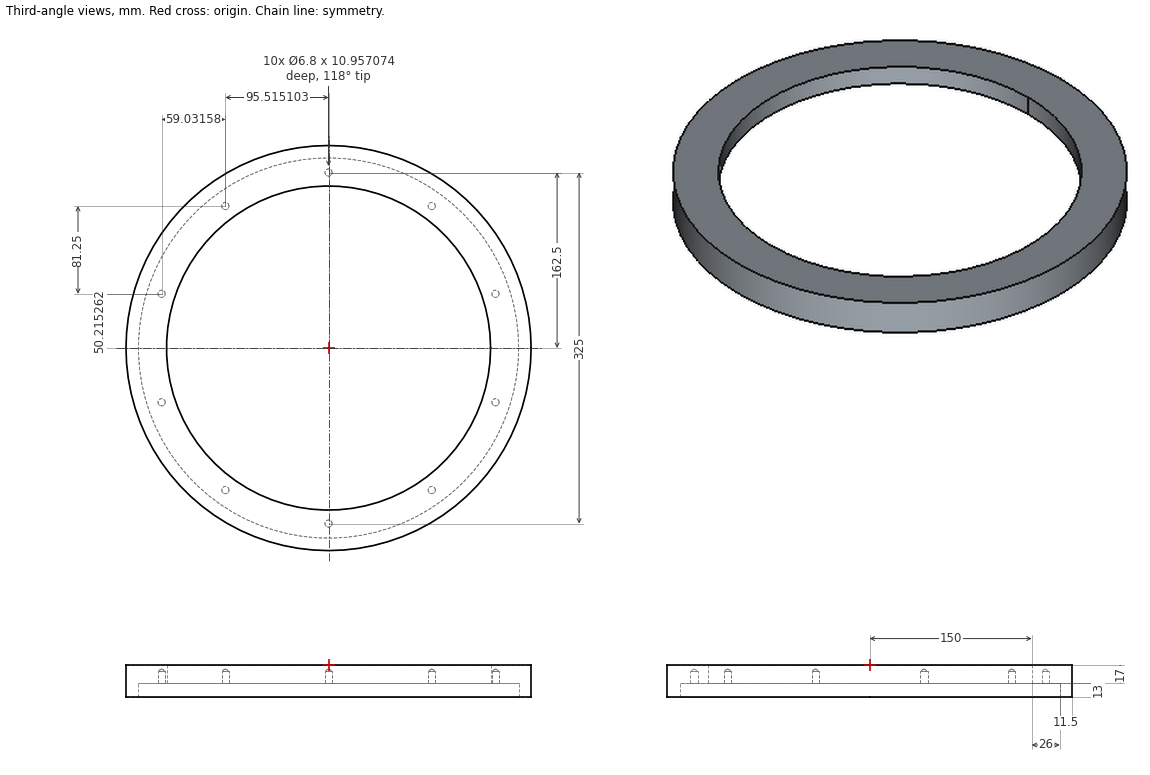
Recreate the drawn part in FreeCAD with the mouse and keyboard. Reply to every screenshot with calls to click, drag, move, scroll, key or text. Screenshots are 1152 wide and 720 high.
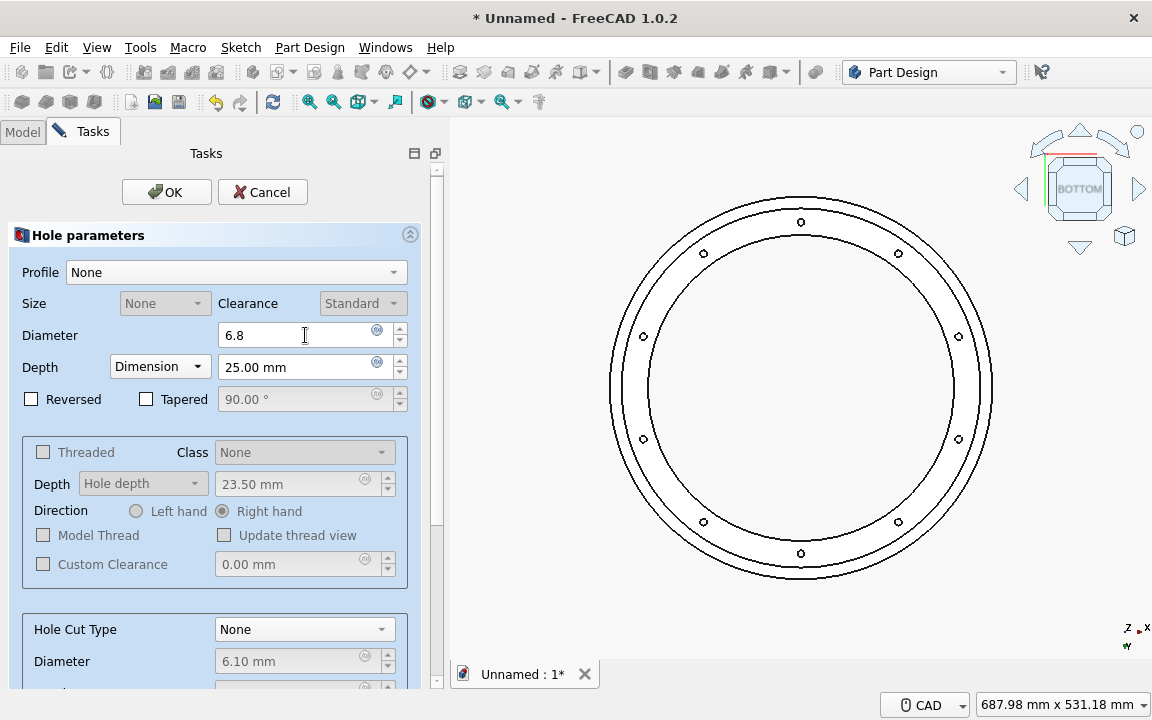
triple_click(305, 367)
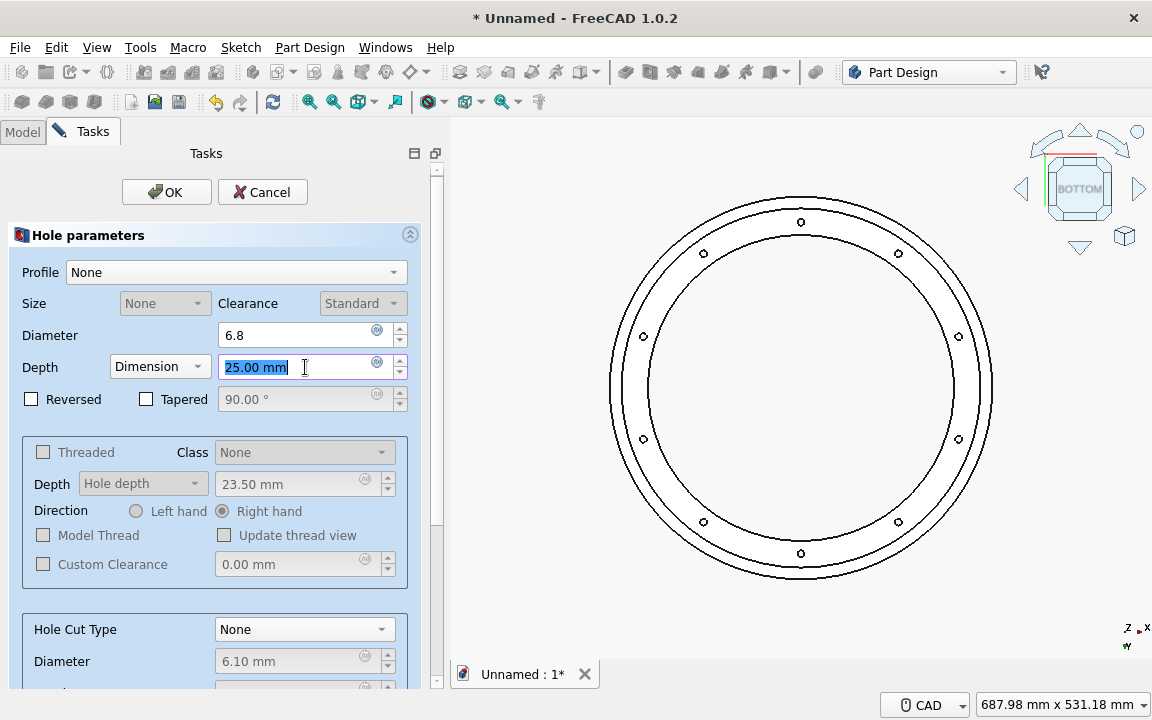
text(10.957074)
key(Tab)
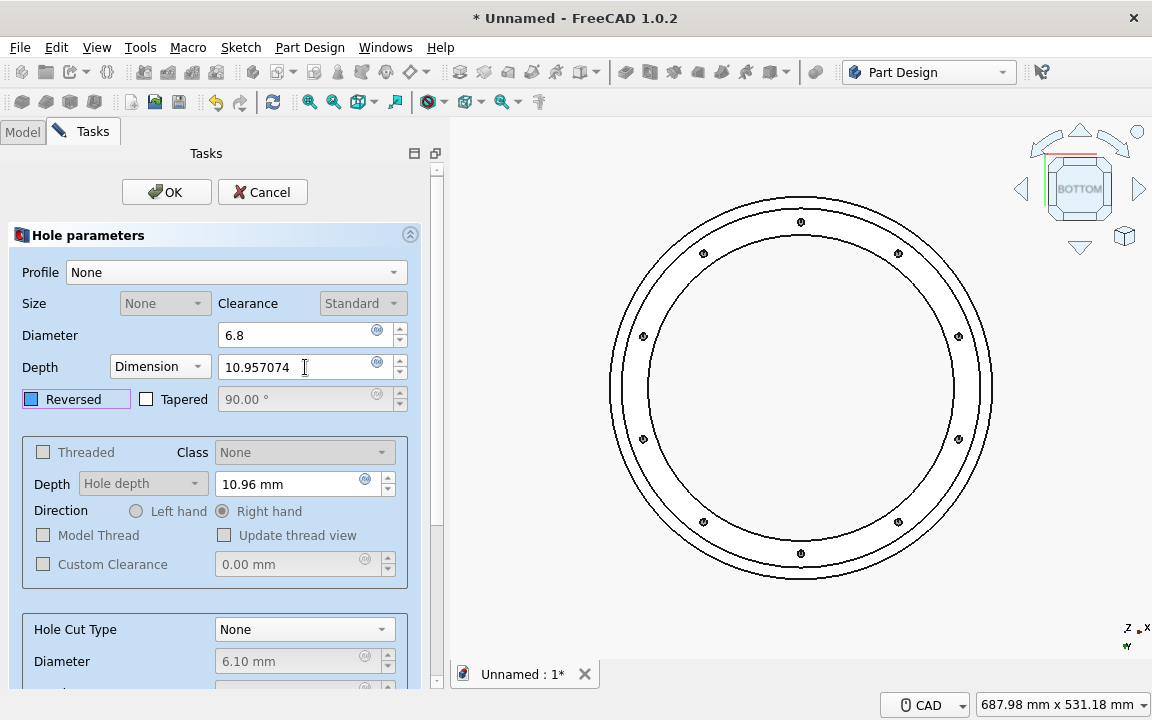
click(167, 192)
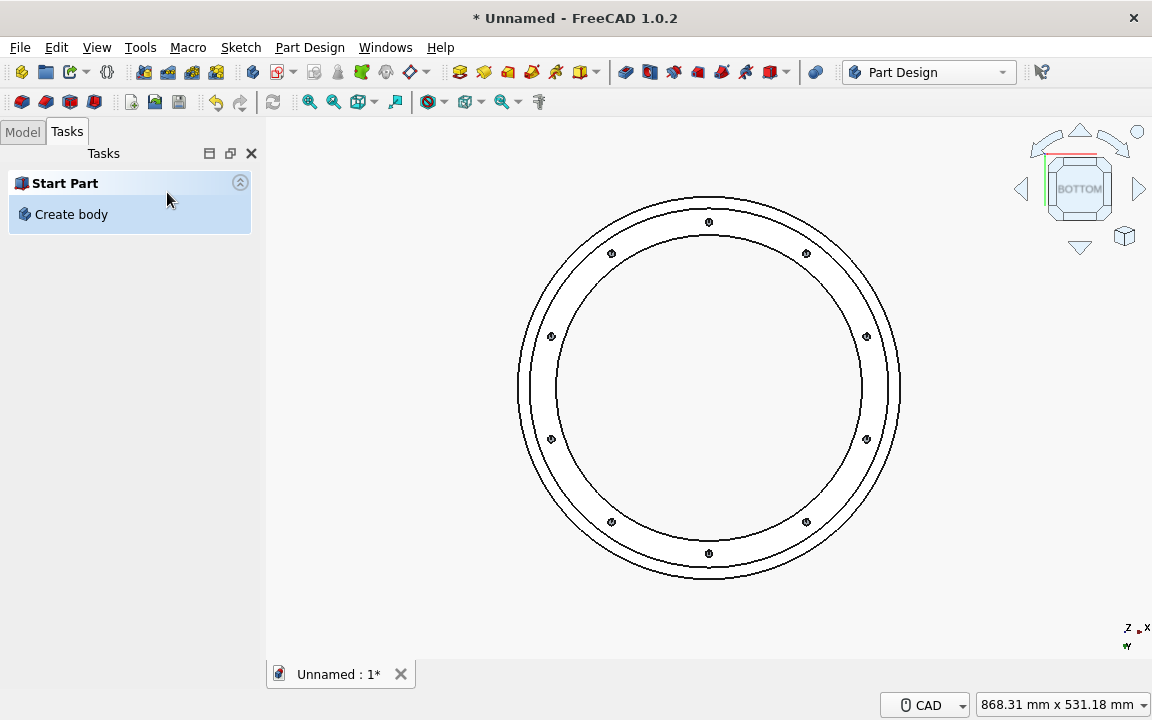
key(0)